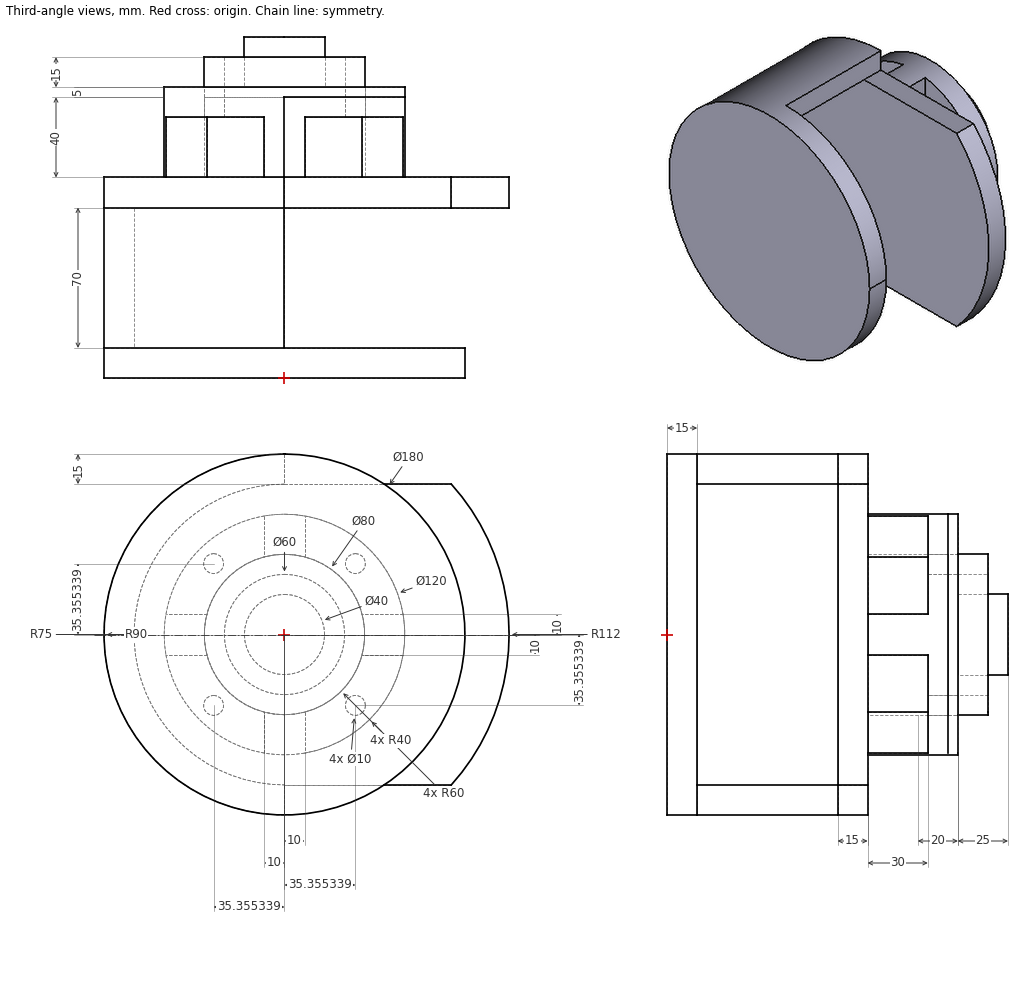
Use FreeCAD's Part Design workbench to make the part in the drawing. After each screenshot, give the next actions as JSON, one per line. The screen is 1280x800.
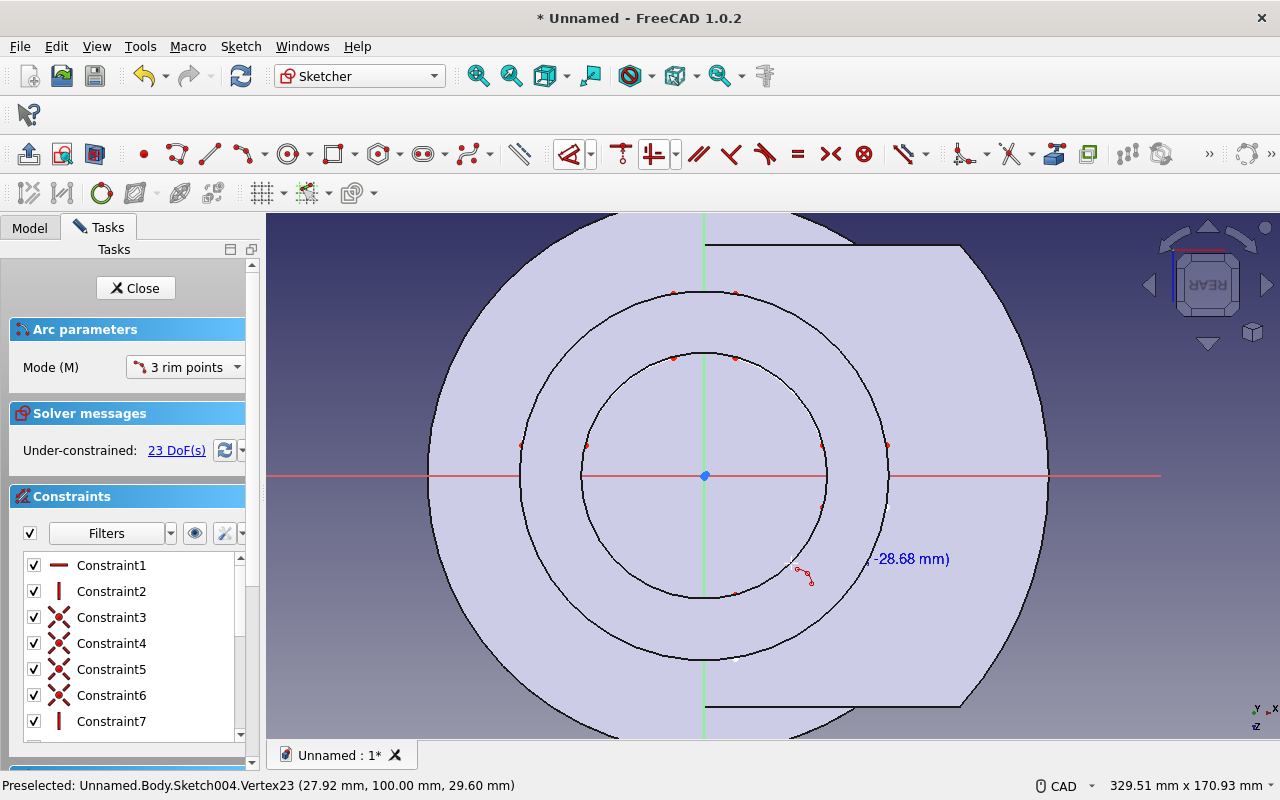
{"action": "left_click", "coordinate": [735, 659]}
{"action": "left_click", "coordinate": [886, 508]}
{"action": "left_click", "coordinate": [835, 606]}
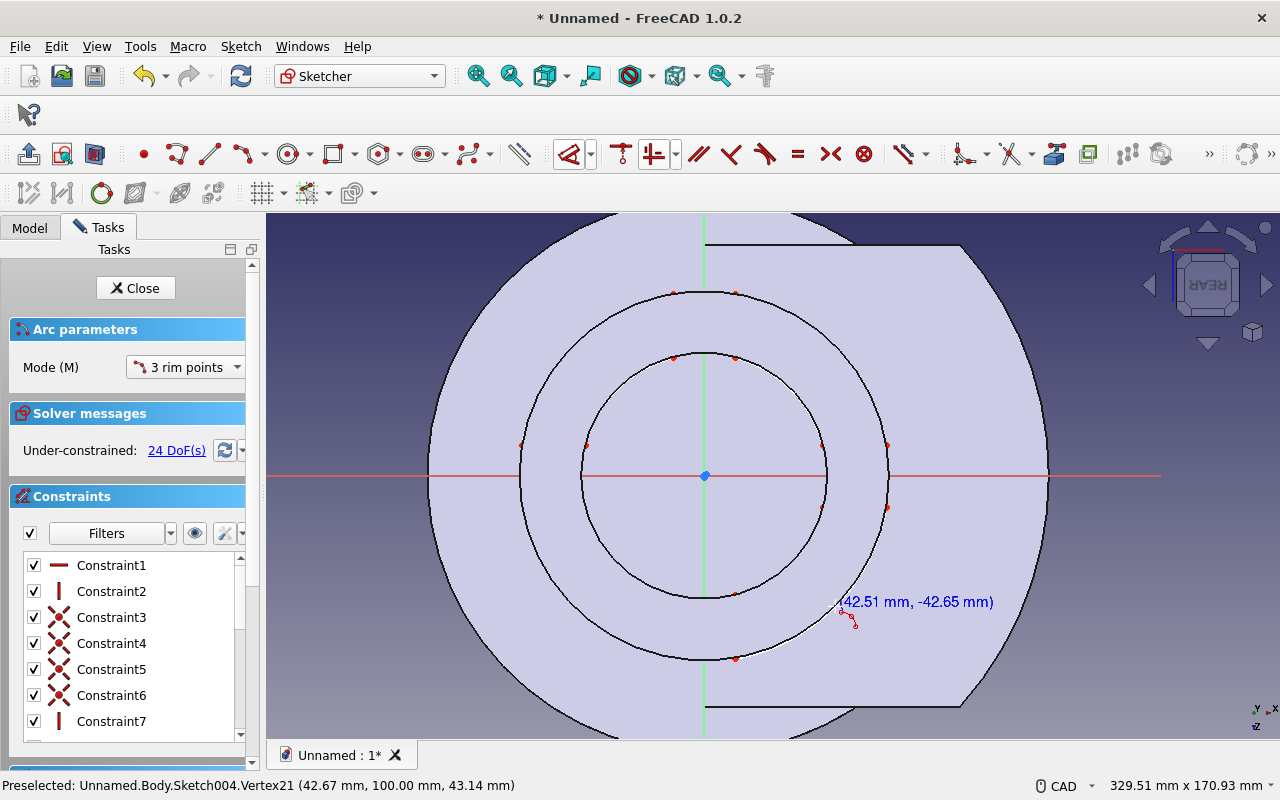
{"action": "left_click", "coordinate": [210, 154]}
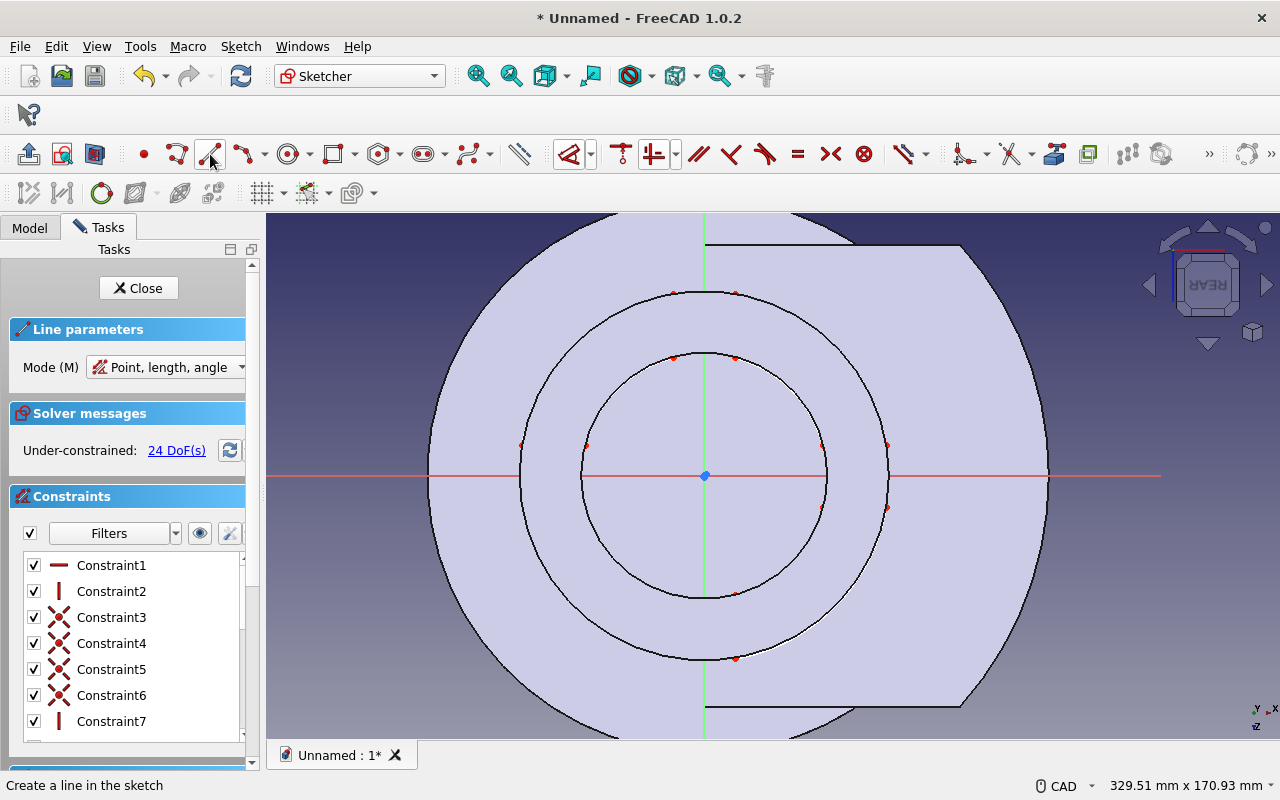
{"action": "left_click", "coordinate": [673, 658]}
{"action": "left_click", "coordinate": [673, 595]}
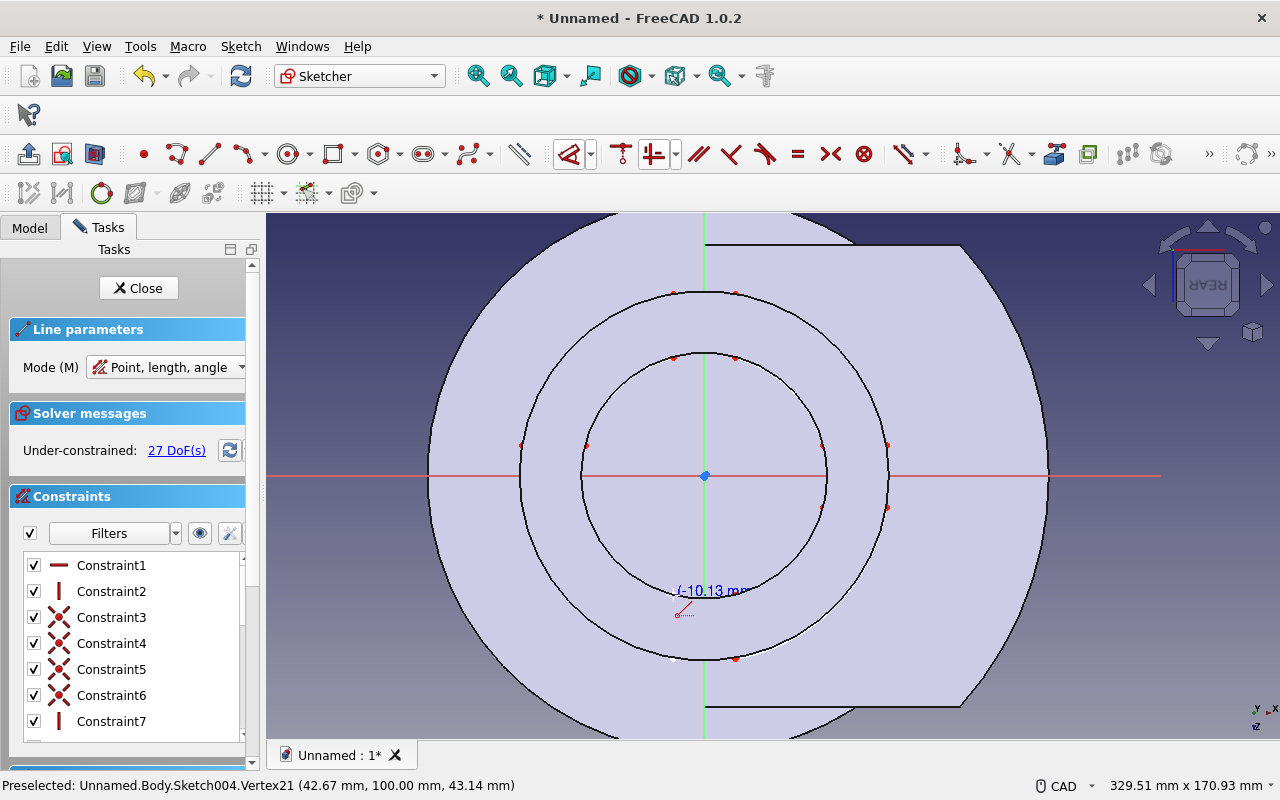
{"action": "left_click", "coordinate": [585, 507]}
{"action": "left_click", "coordinate": [522, 507]}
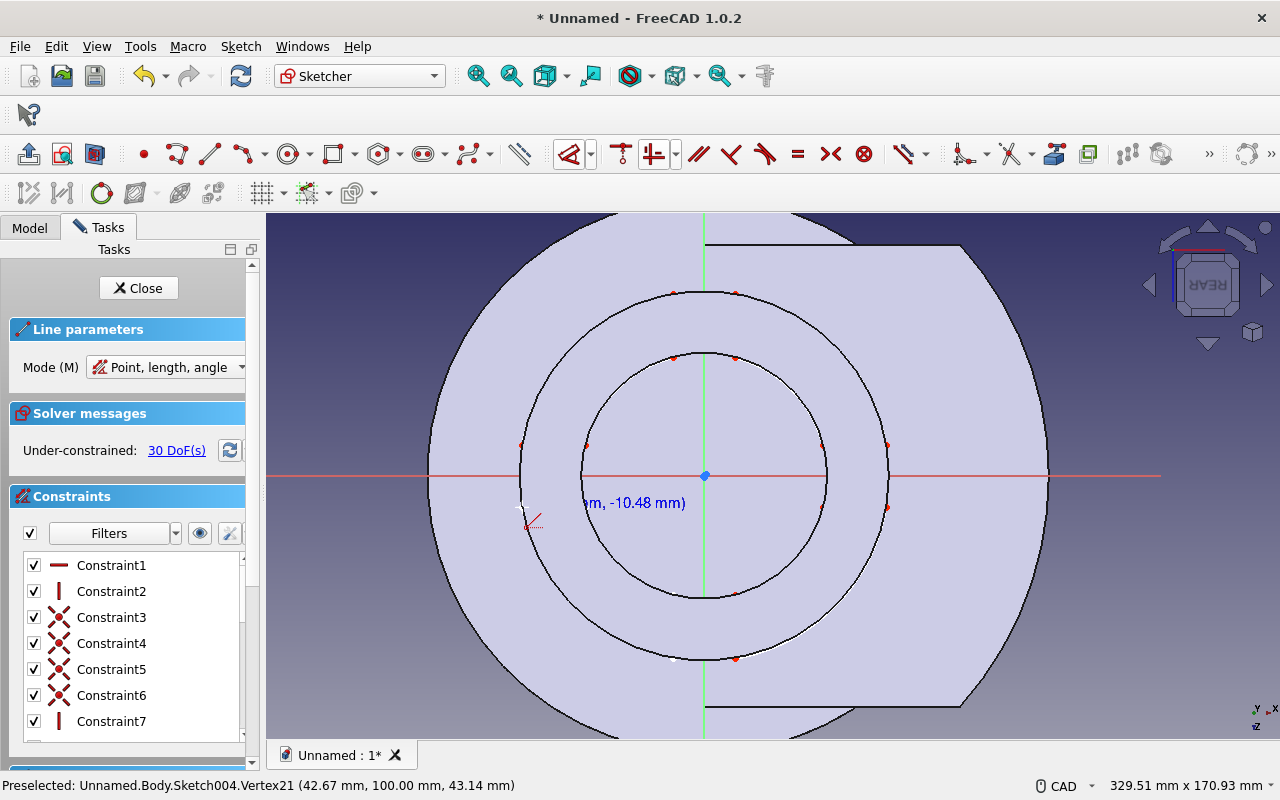
{"action": "left_click", "coordinate": [242, 154]}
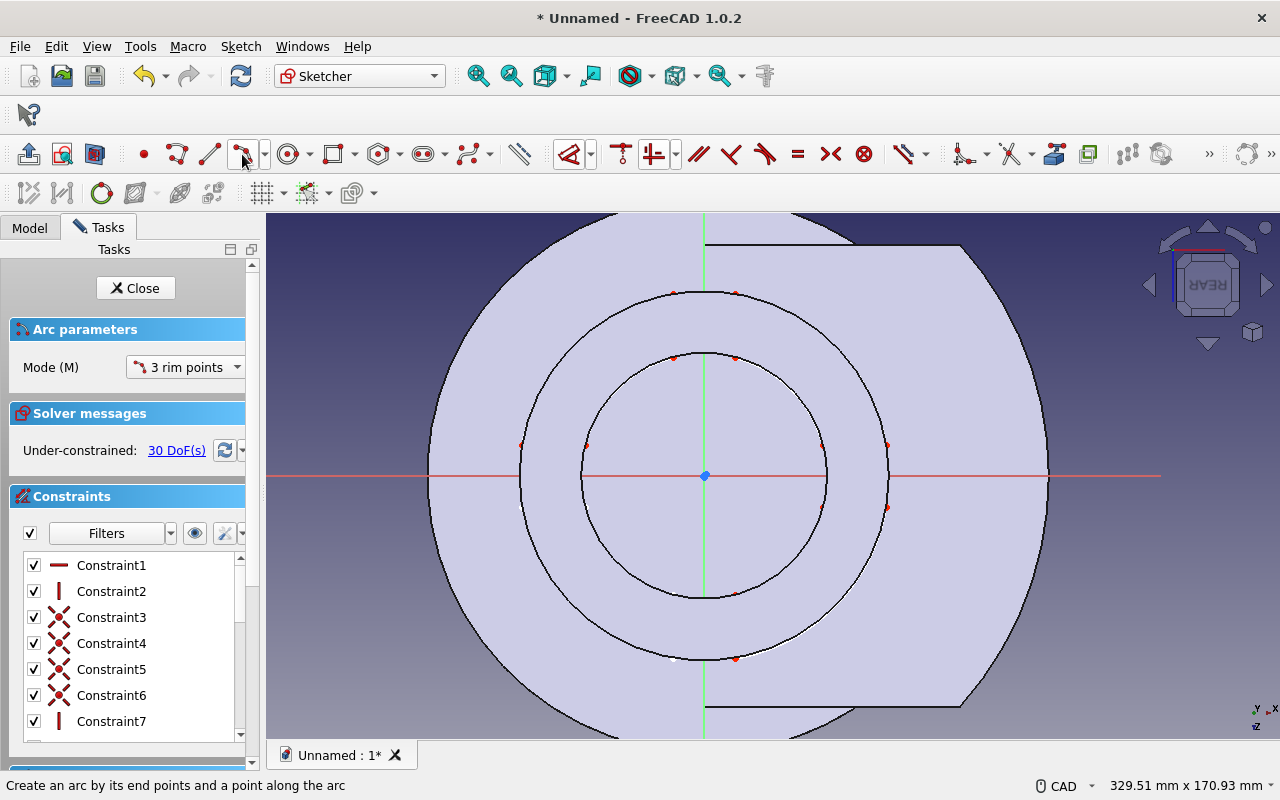
{"action": "left_click", "coordinate": [673, 596]}
{"action": "left_click", "coordinate": [585, 508]}
{"action": "left_click", "coordinate": [617, 563]}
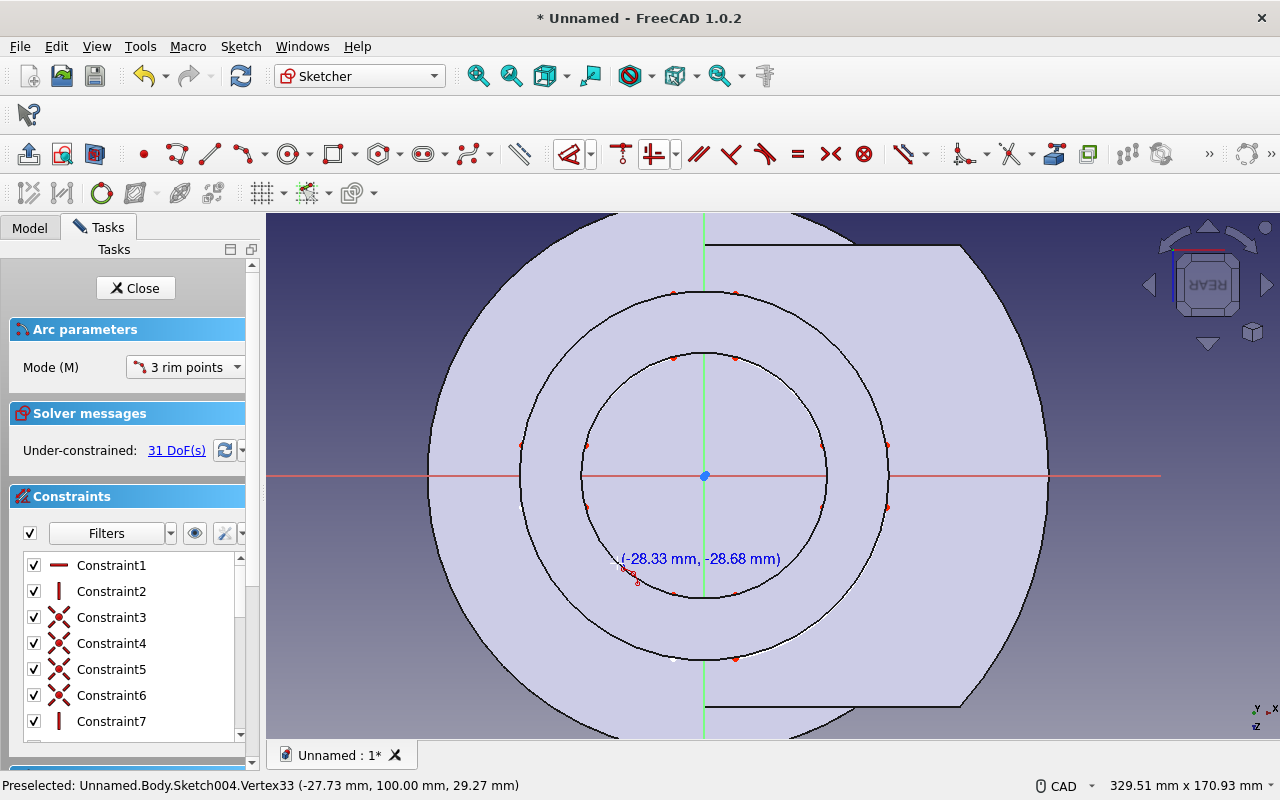
{"action": "left_click", "coordinate": [522, 508]}
{"action": "left_click", "coordinate": [673, 659]}
{"action": "left_click", "coordinate": [574, 606]}
{"action": "key", "text": "Escape"}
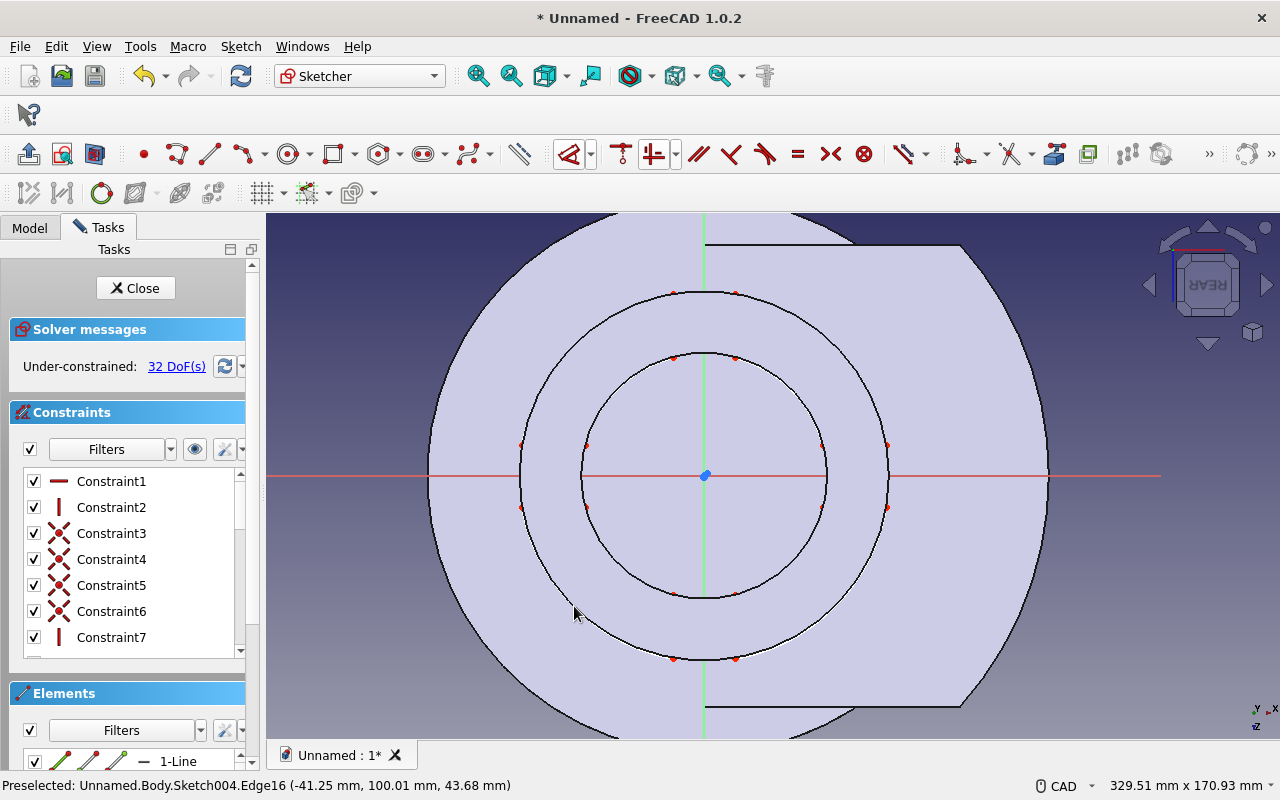
{"action": "left_click", "coordinate": [863, 382]}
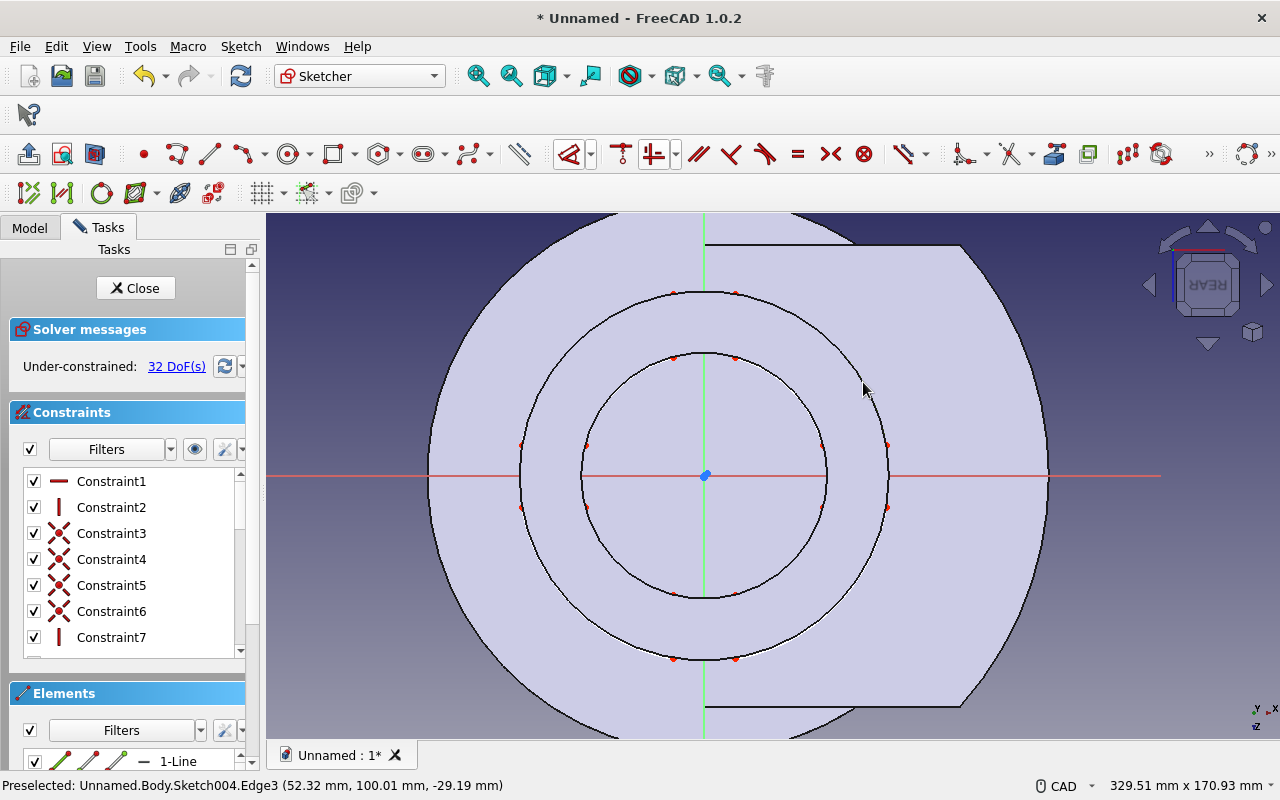
{"action": "left_click", "coordinate": [807, 410]}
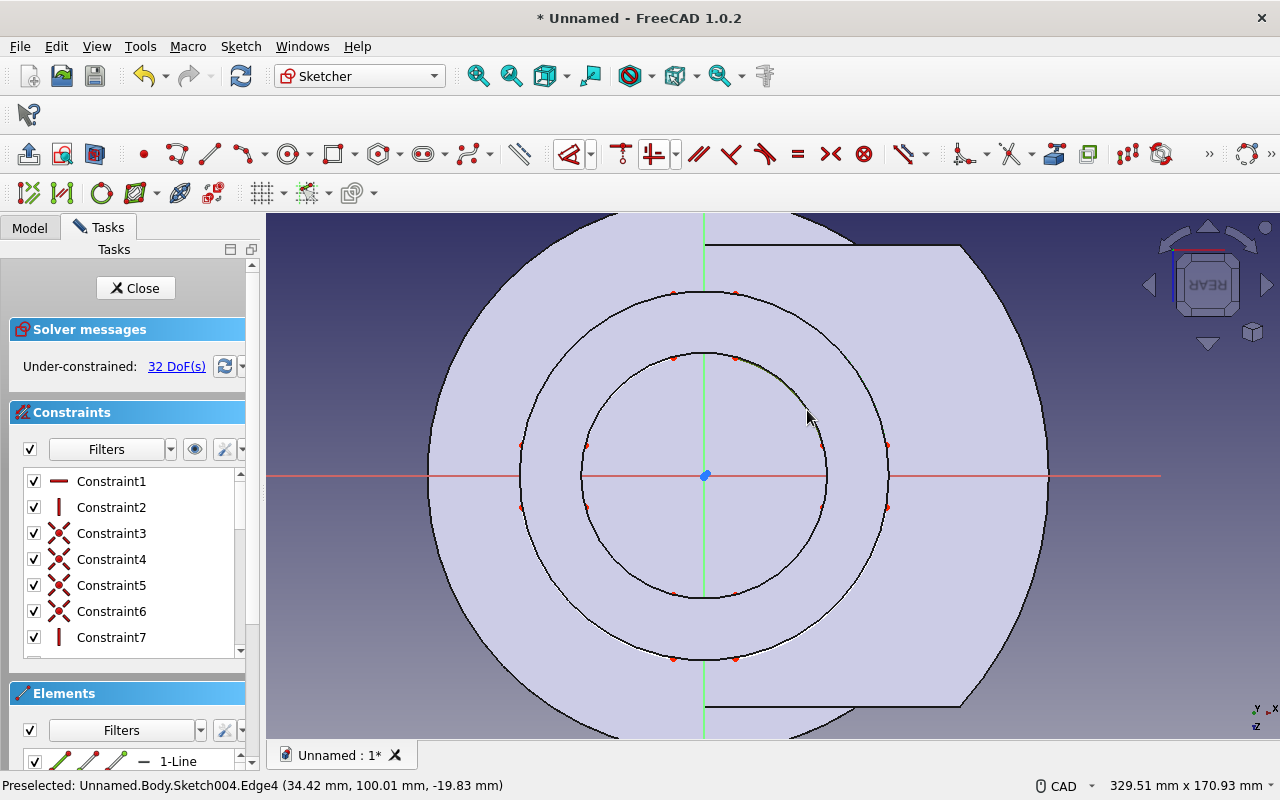
{"action": "left_click", "coordinate": [621, 154]}